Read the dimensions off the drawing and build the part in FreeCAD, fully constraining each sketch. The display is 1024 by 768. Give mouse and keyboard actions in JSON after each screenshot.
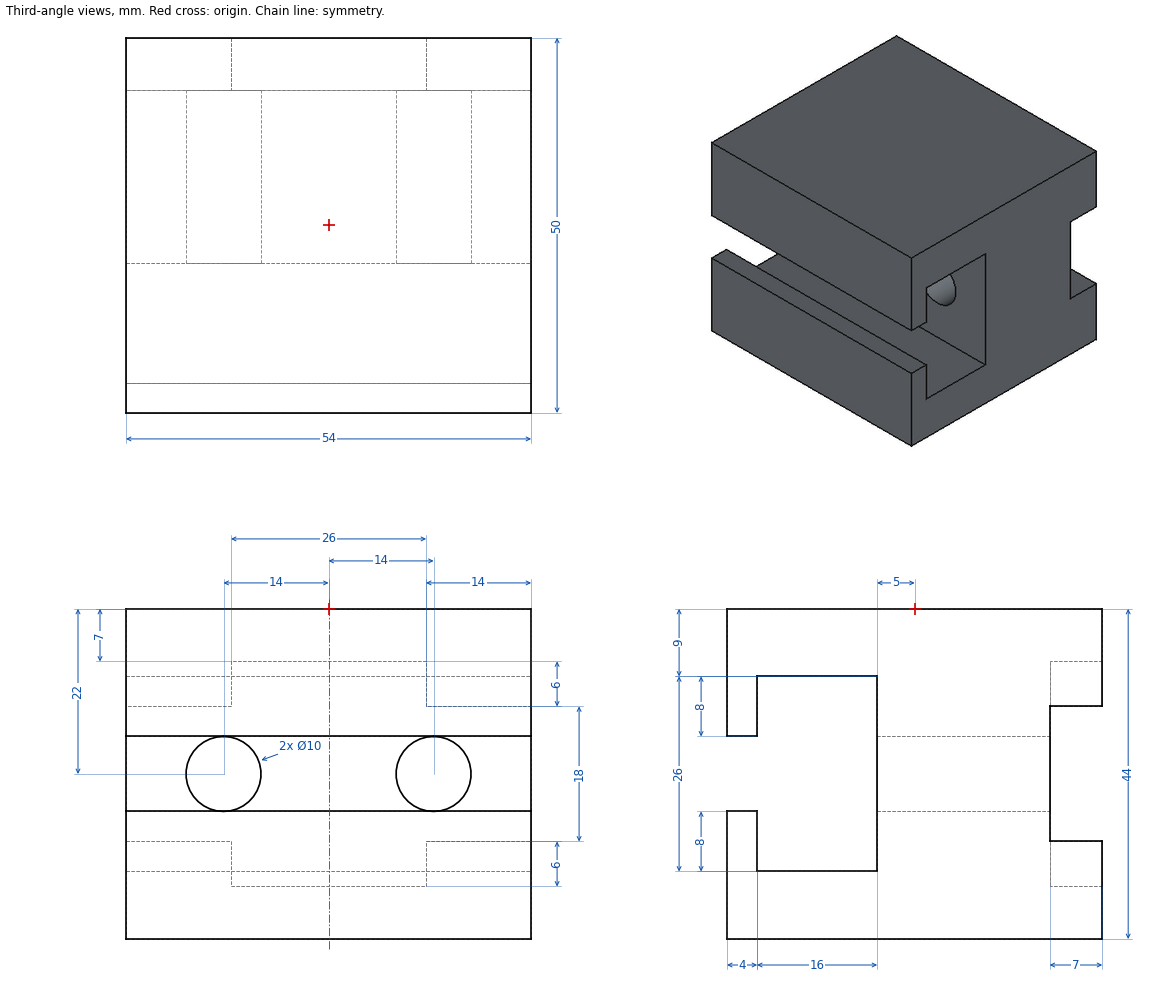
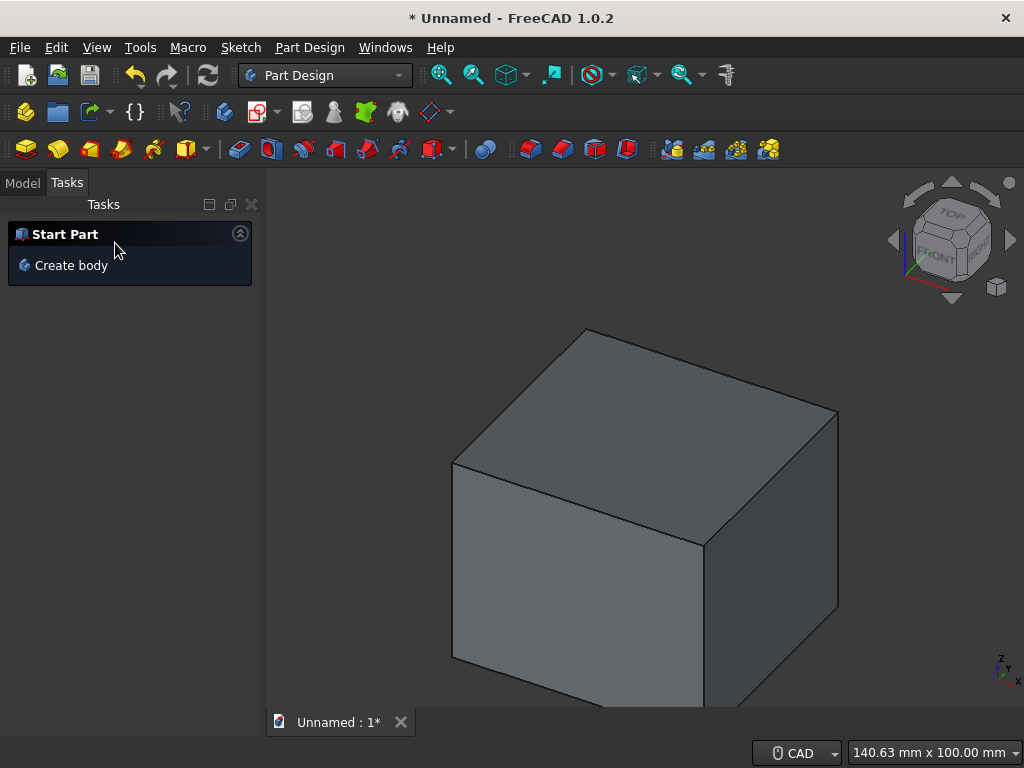
{"action": "key", "text": "v f"}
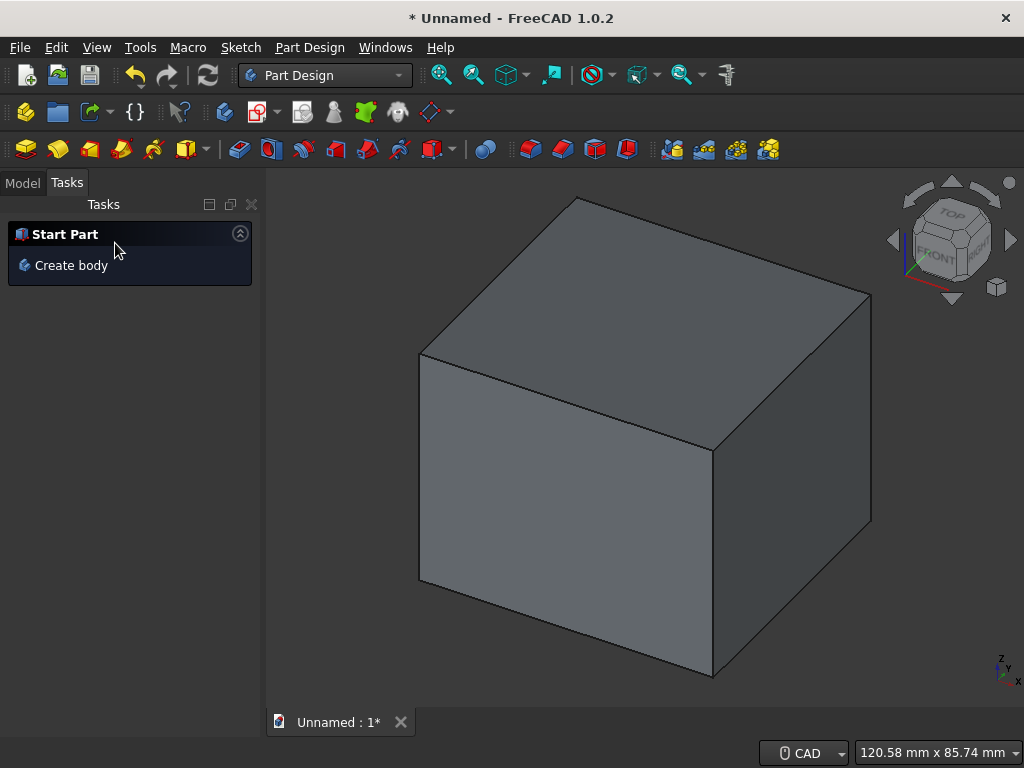
{"action": "key", "text": "4"}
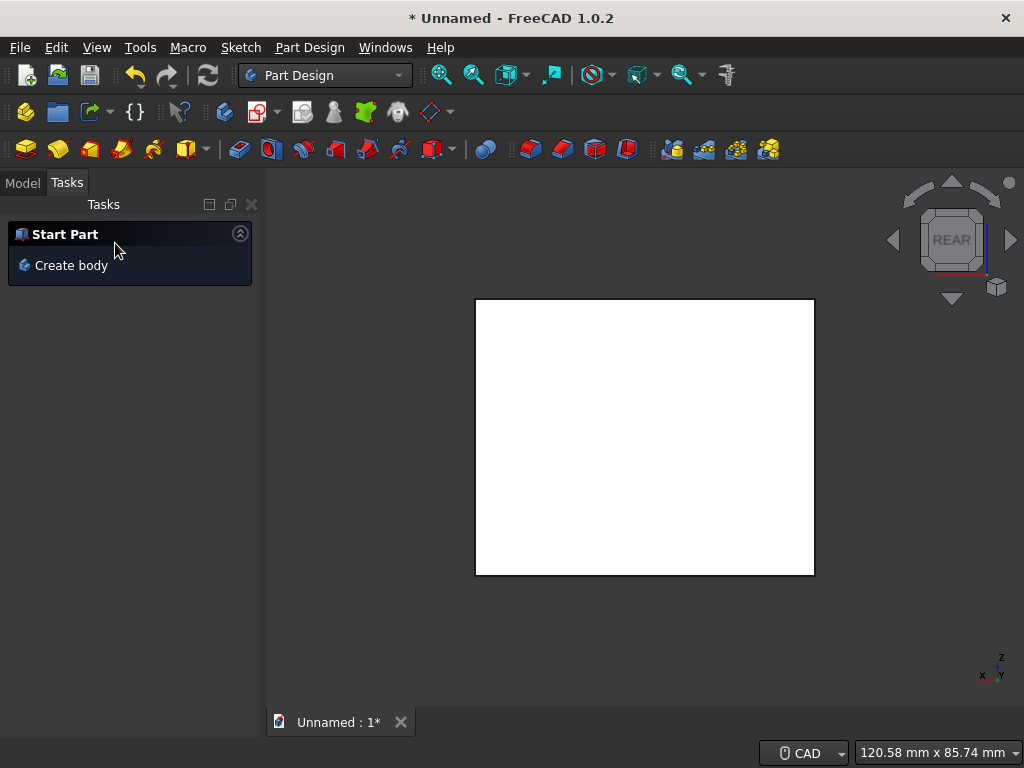
{"action": "left_click", "coordinate": [645, 437]}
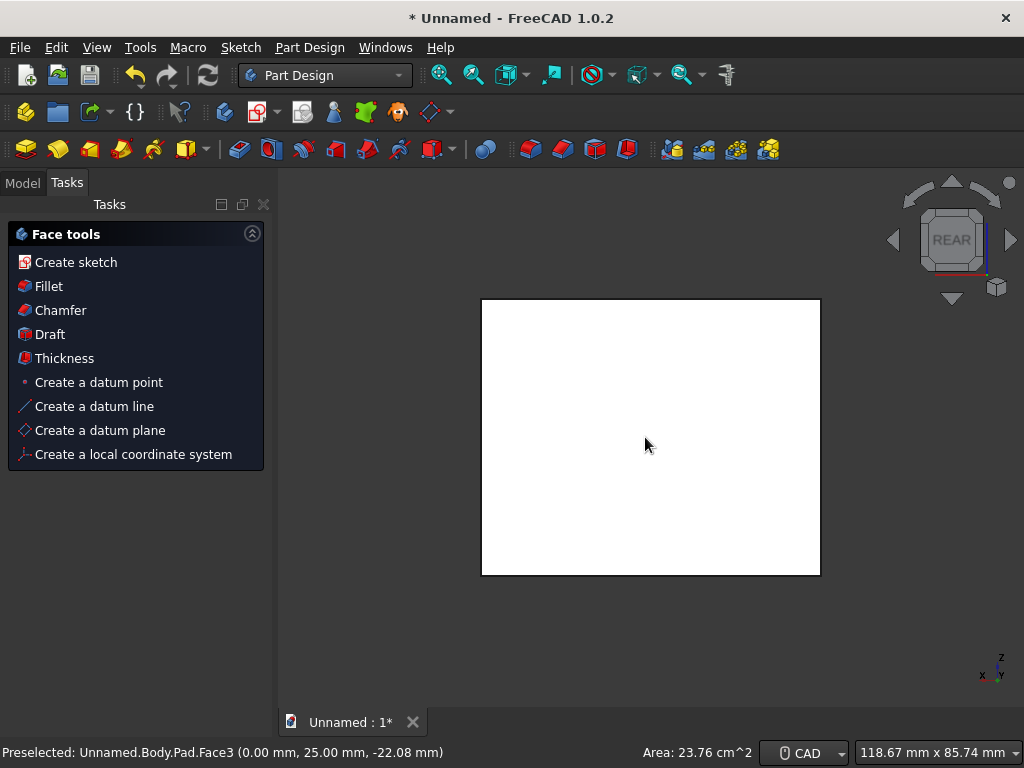
{"action": "left_click", "coordinate": [258, 112]}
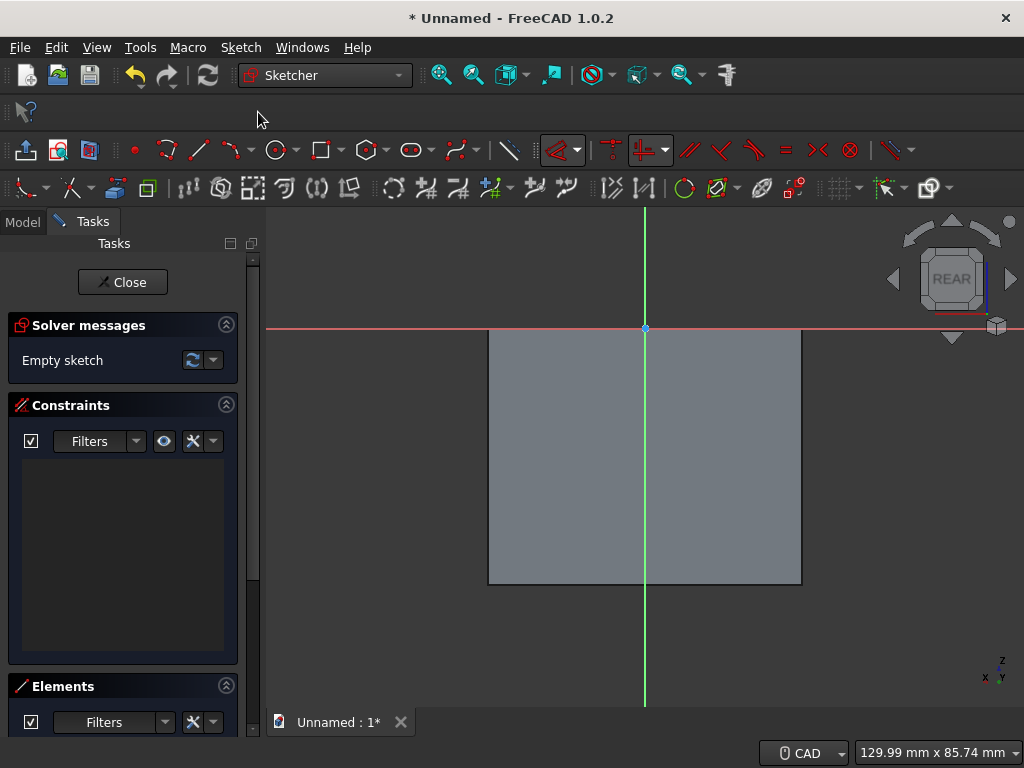
{"action": "key", "text": "g m"}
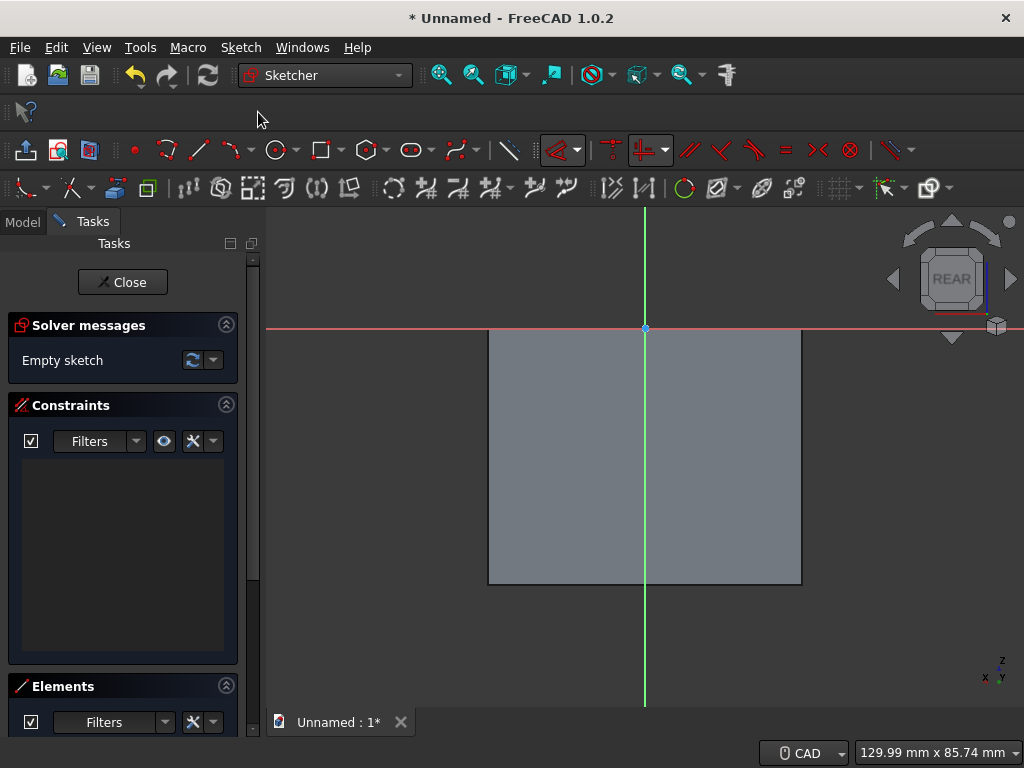
{"action": "left_click", "coordinate": [721, 370]}
{"action": "left_click", "coordinate": [569, 370]}
{"action": "left_click", "coordinate": [569, 405]}
{"action": "left_click", "coordinate": [488, 405]}
{"action": "left_click", "coordinate": [488, 509]}
{"action": "left_click", "coordinate": [569, 509]}
{"action": "left_click", "coordinate": [569, 544]}
{"action": "left_click", "coordinate": [721, 544]}
{"action": "left_click", "coordinate": [721, 509]}
{"action": "left_click", "coordinate": [802, 509]}
{"action": "left_click", "coordinate": [802, 405]}
{"action": "left_click", "coordinate": [721, 405]}
{"action": "left_click", "coordinate": [721, 371]}
{"action": "key", "text": "Escape"}
{"action": "key", "text": "Escape"}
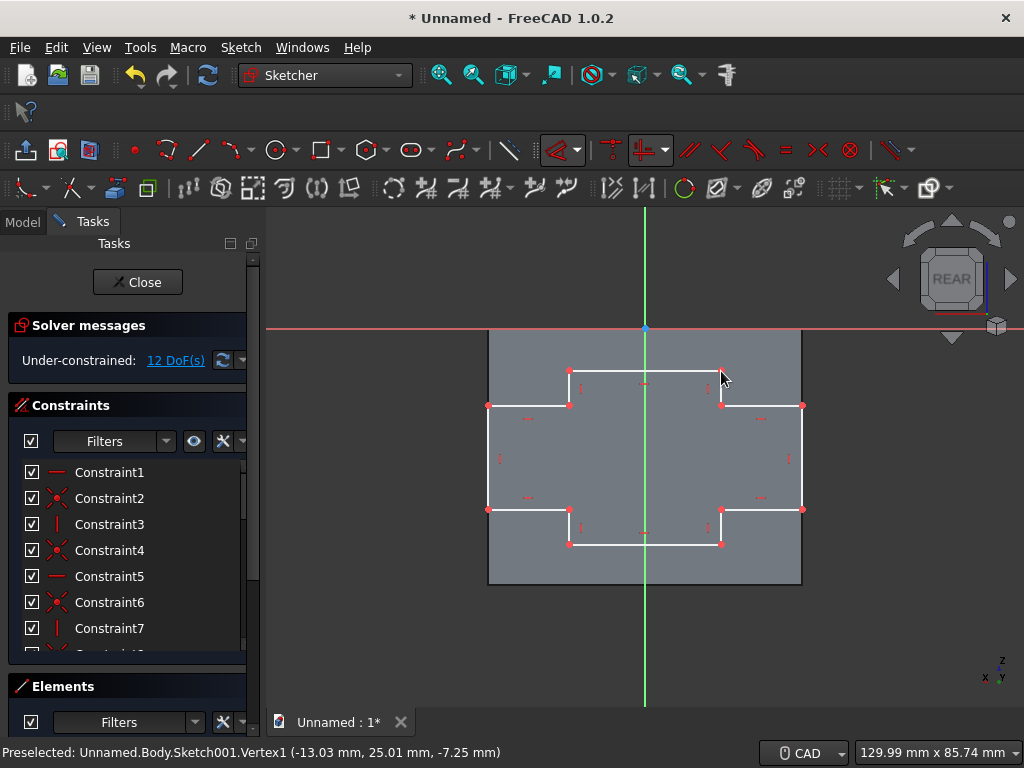
{"action": "left_click", "coordinate": [569, 510]}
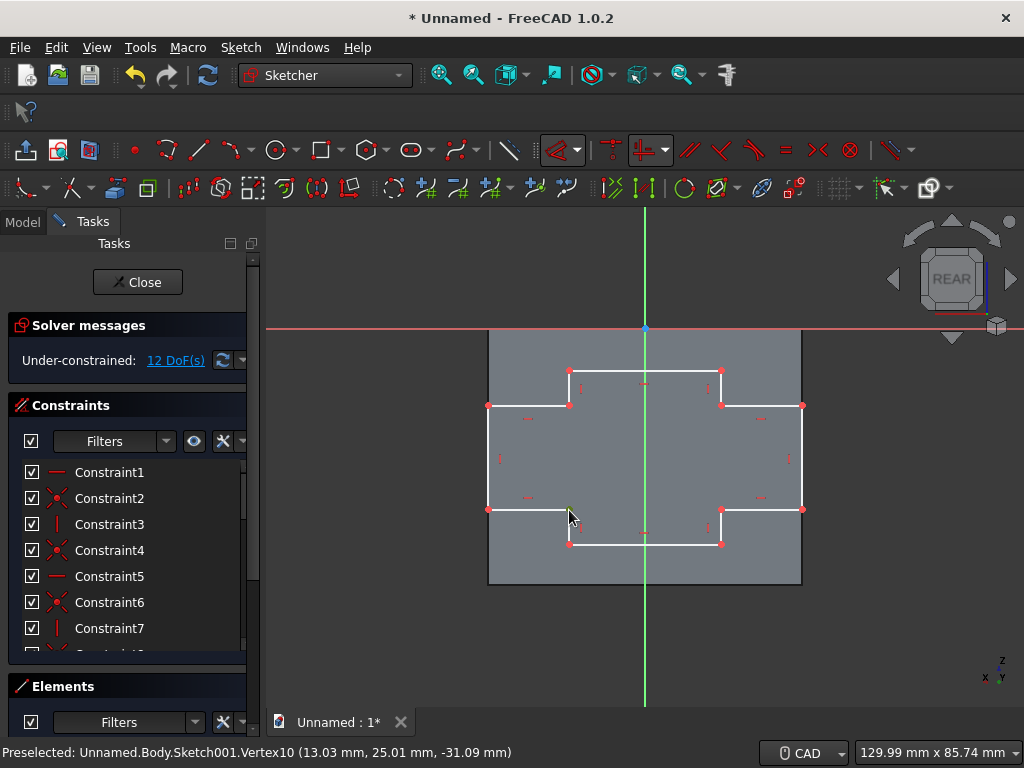
{"action": "left_click", "coordinate": [721, 510]}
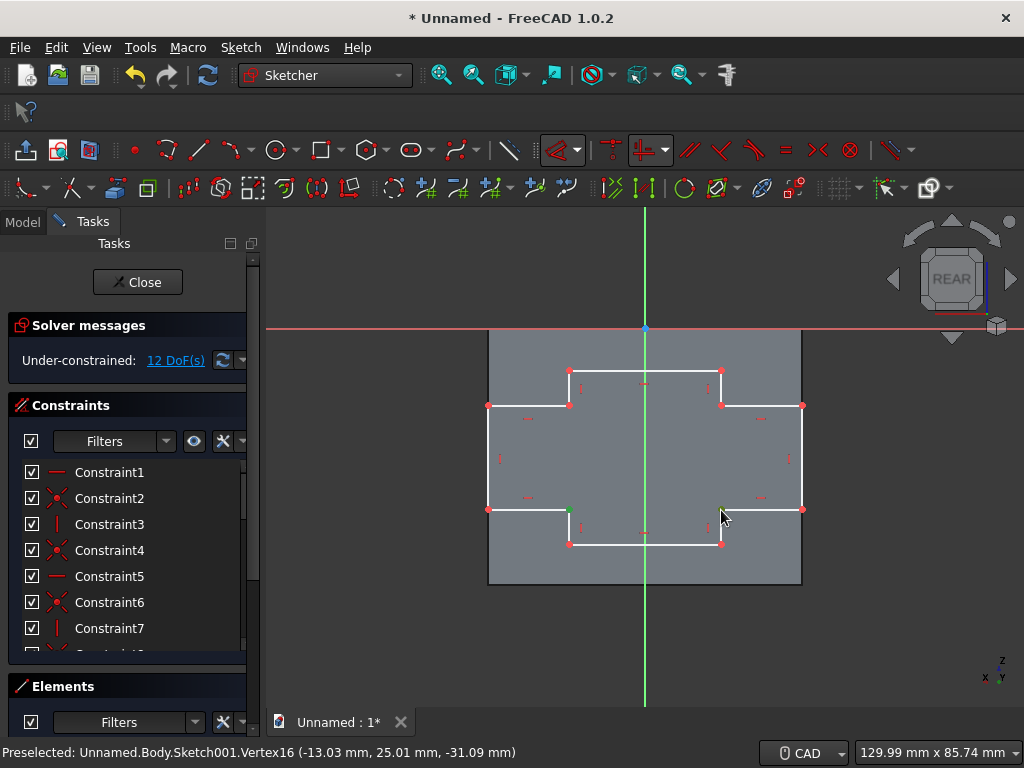
{"action": "left_click", "coordinate": [645, 647]}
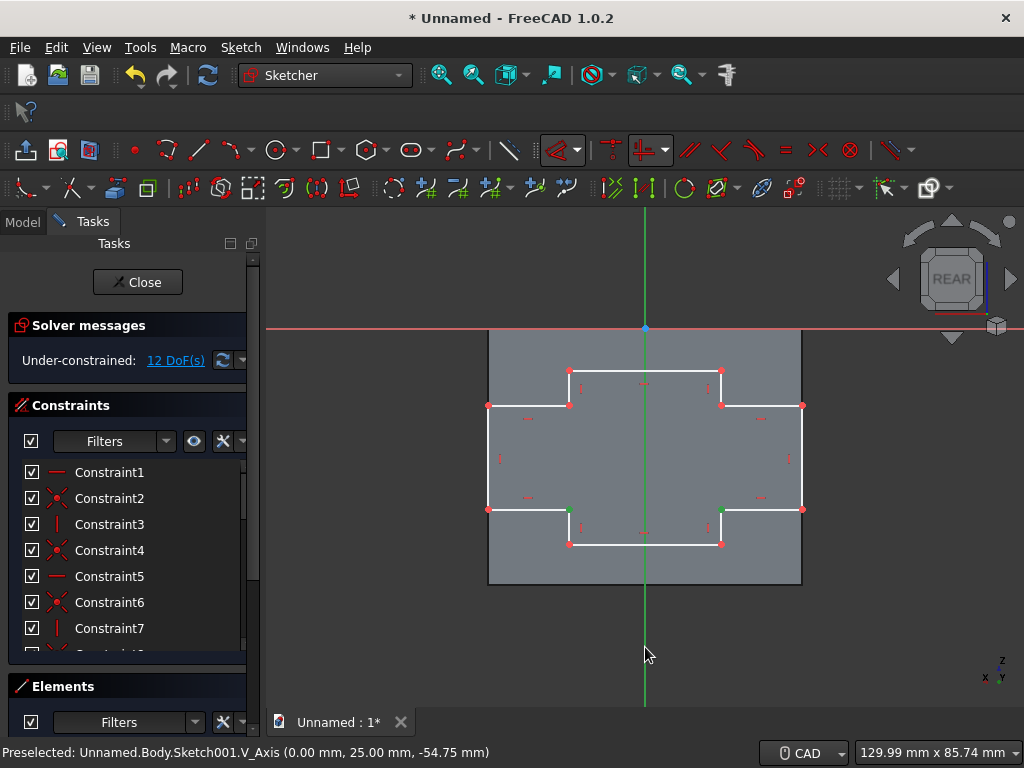
{"action": "key", "text": "s"}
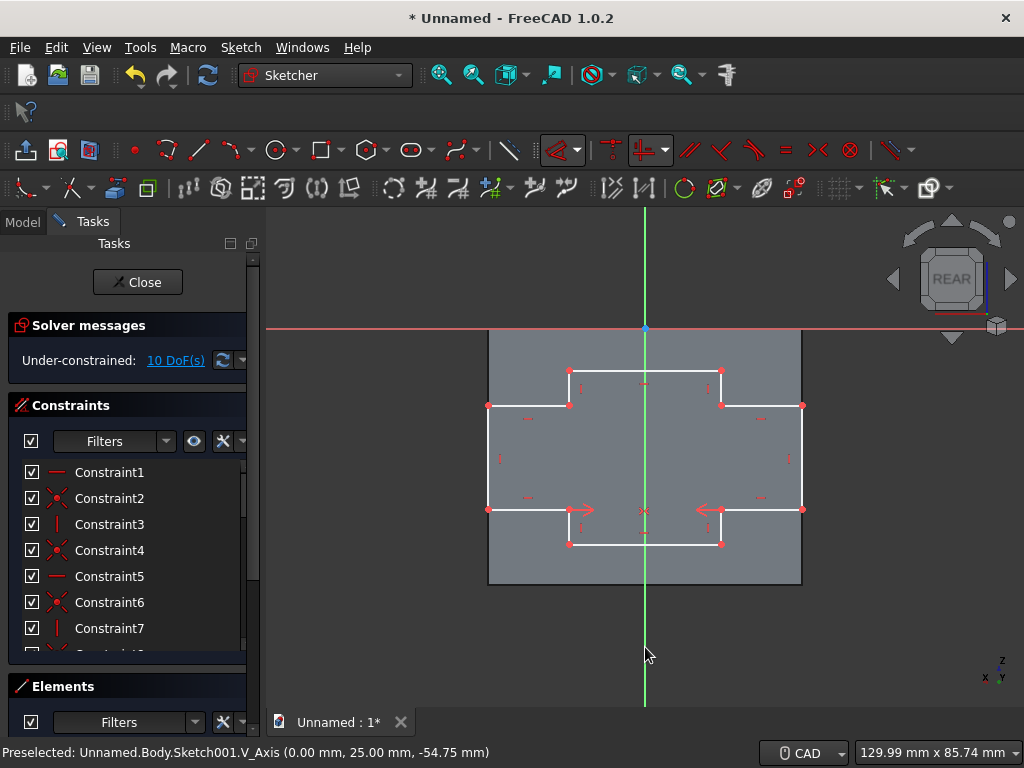
{"action": "left_click", "coordinate": [488, 406]}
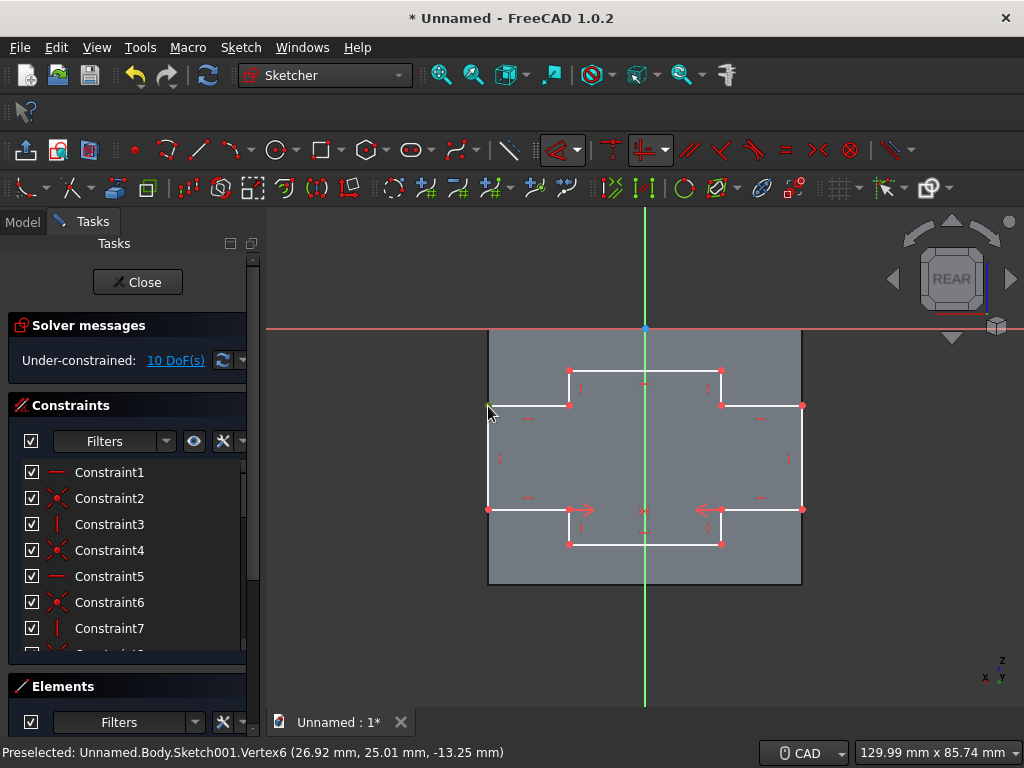
{"action": "left_click", "coordinate": [802, 406]}